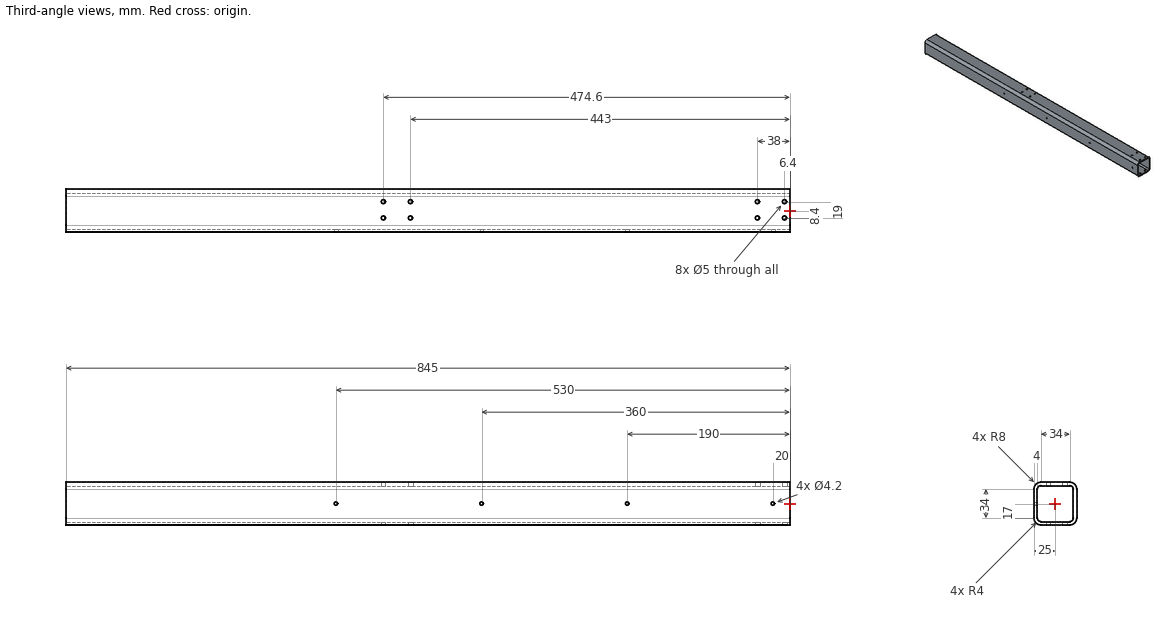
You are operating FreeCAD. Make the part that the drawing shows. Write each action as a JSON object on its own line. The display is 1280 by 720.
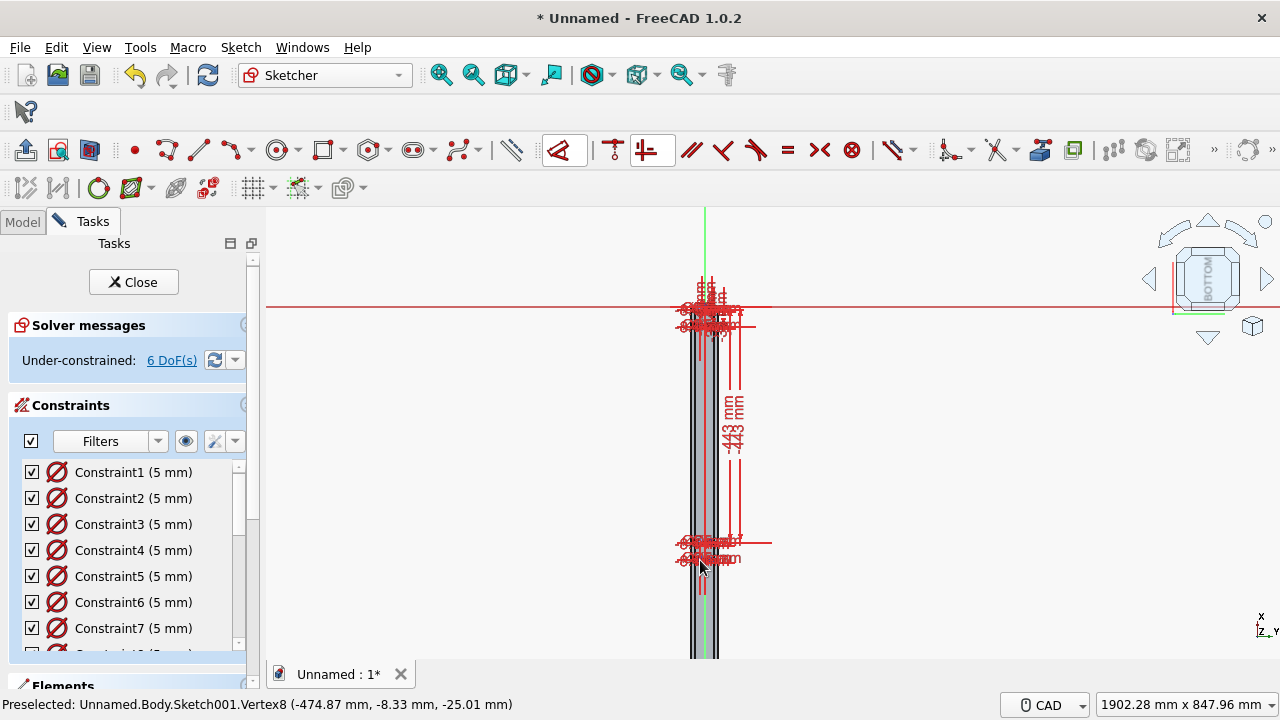
{"action": "scroll", "coordinate": [710, 310], "scroll_direction": "up", "scroll_amount": 7}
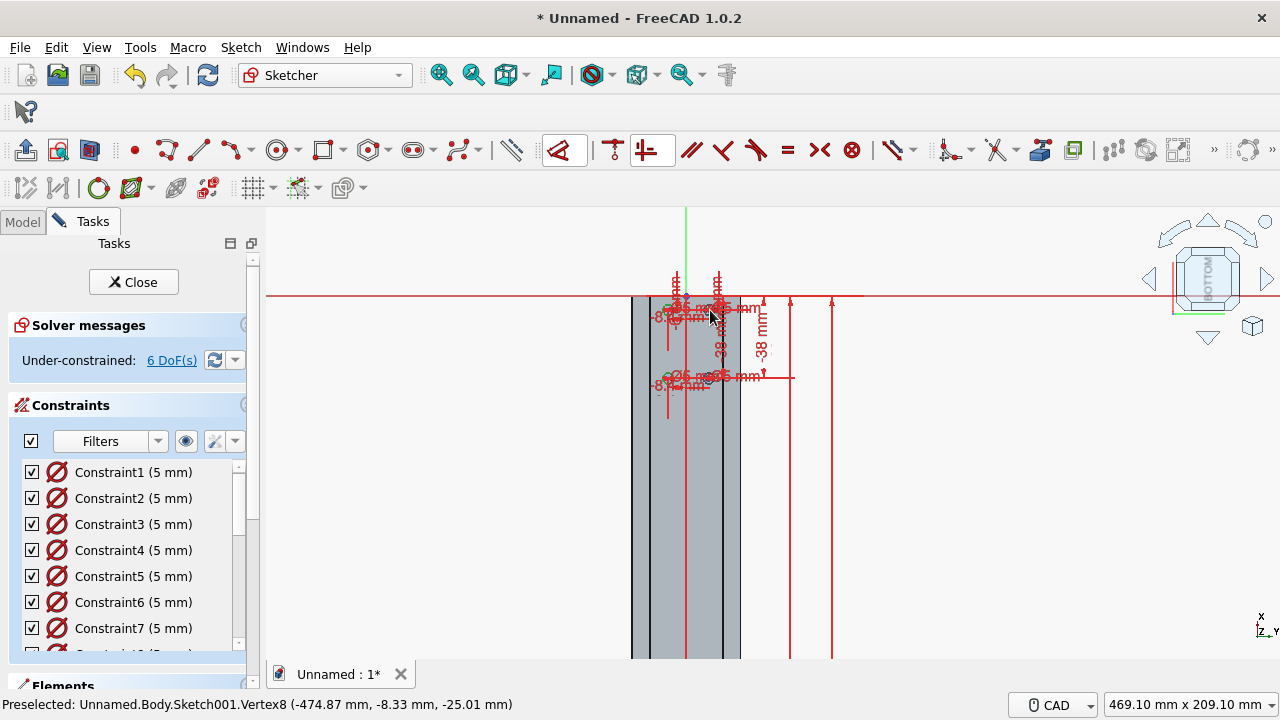
{"action": "left_click", "coordinate": [710, 310]}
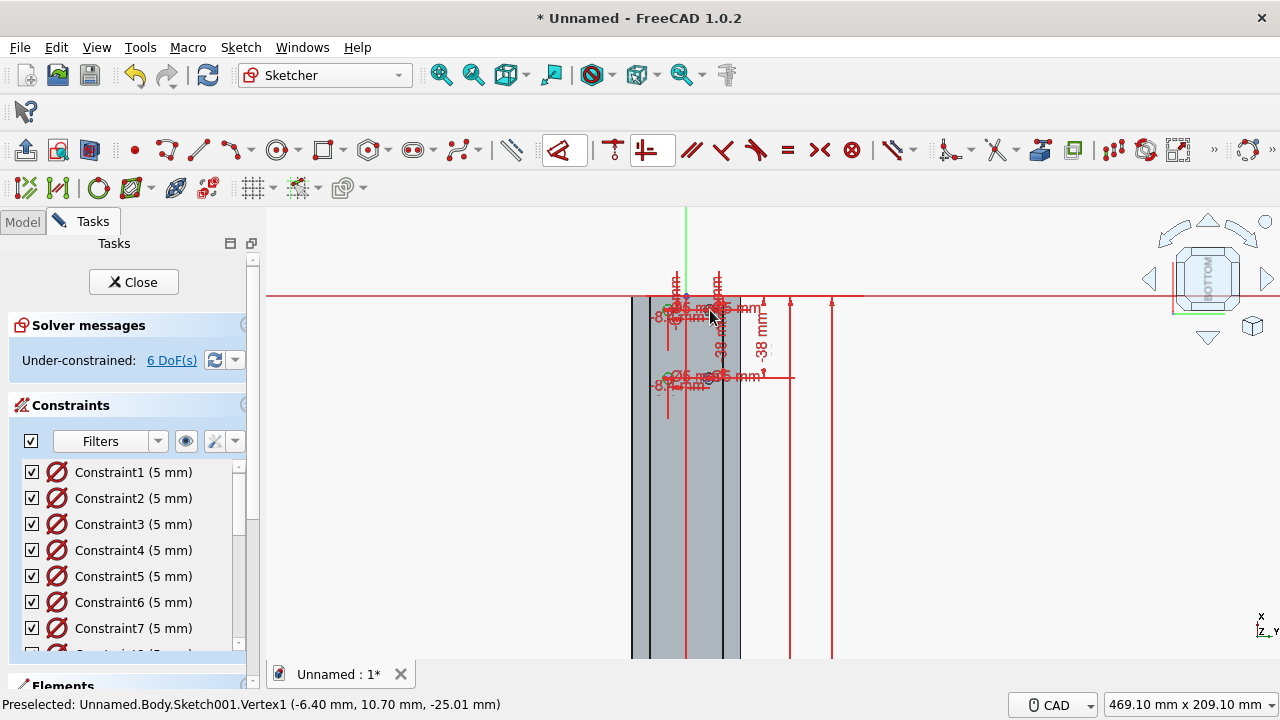
{"action": "left_click", "coordinate": [668, 310]}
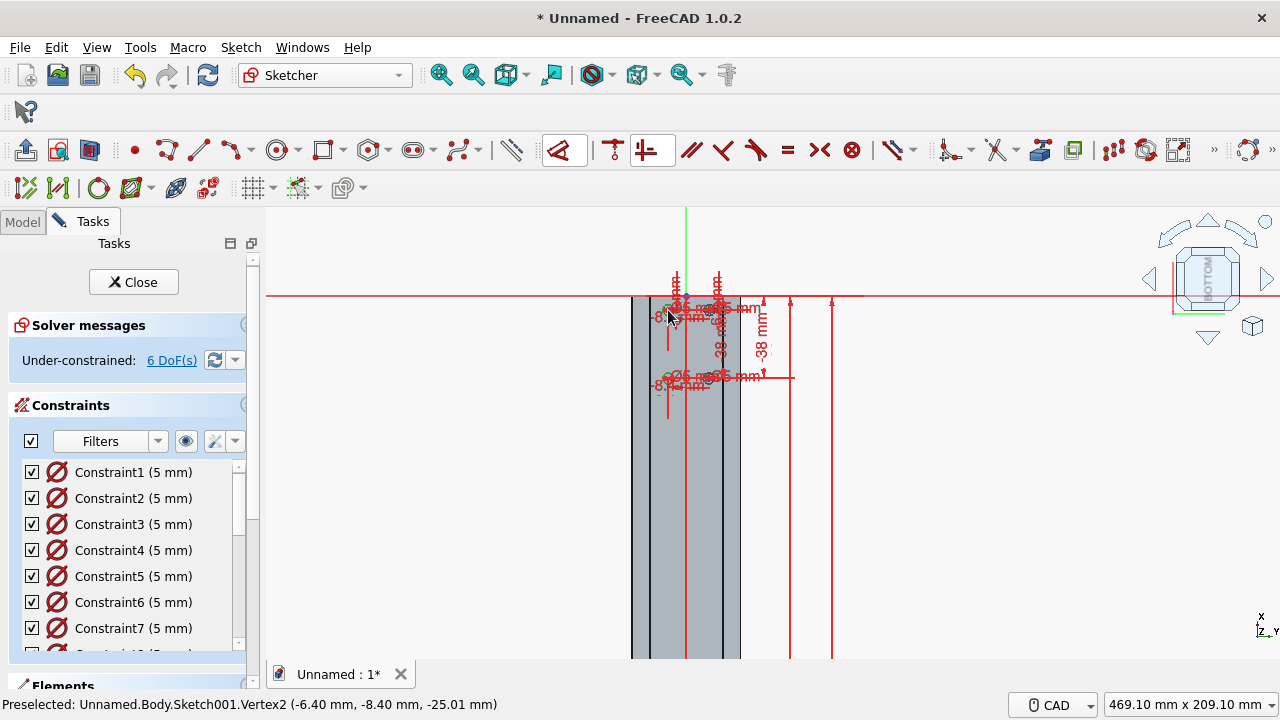
{"action": "left_click", "coordinate": [582, 150]}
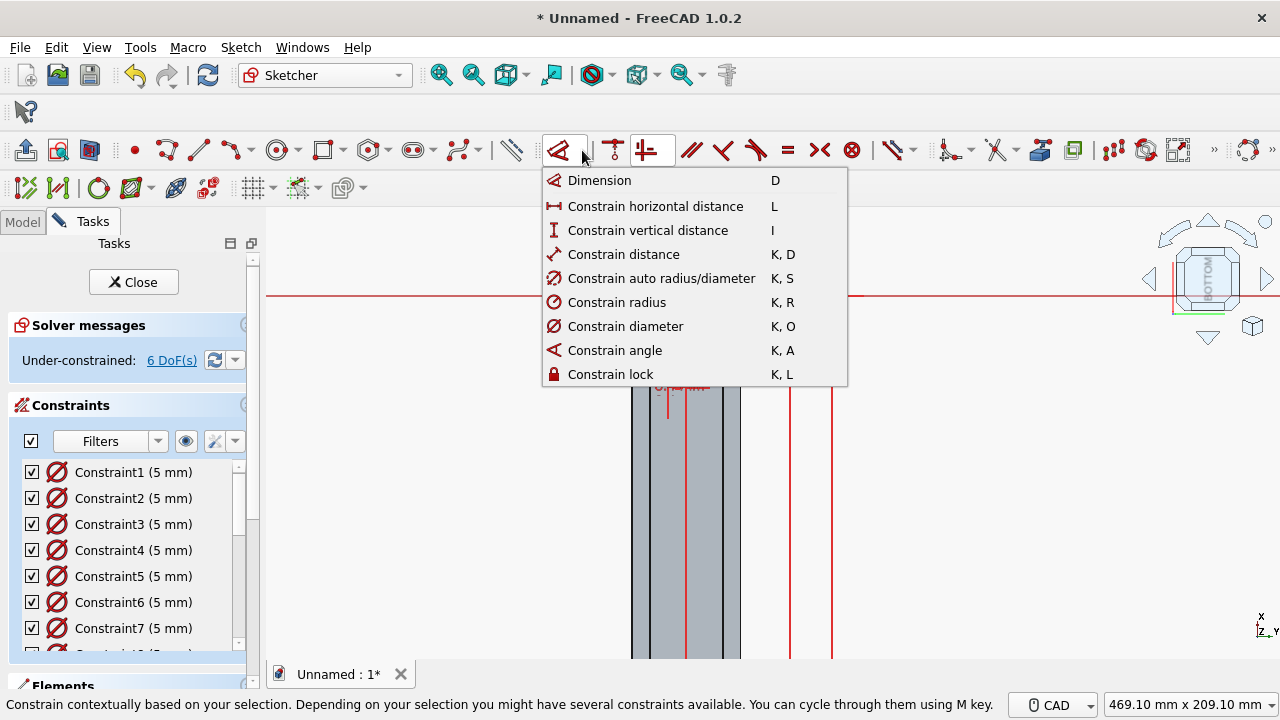
{"action": "left_click", "coordinate": [695, 206]}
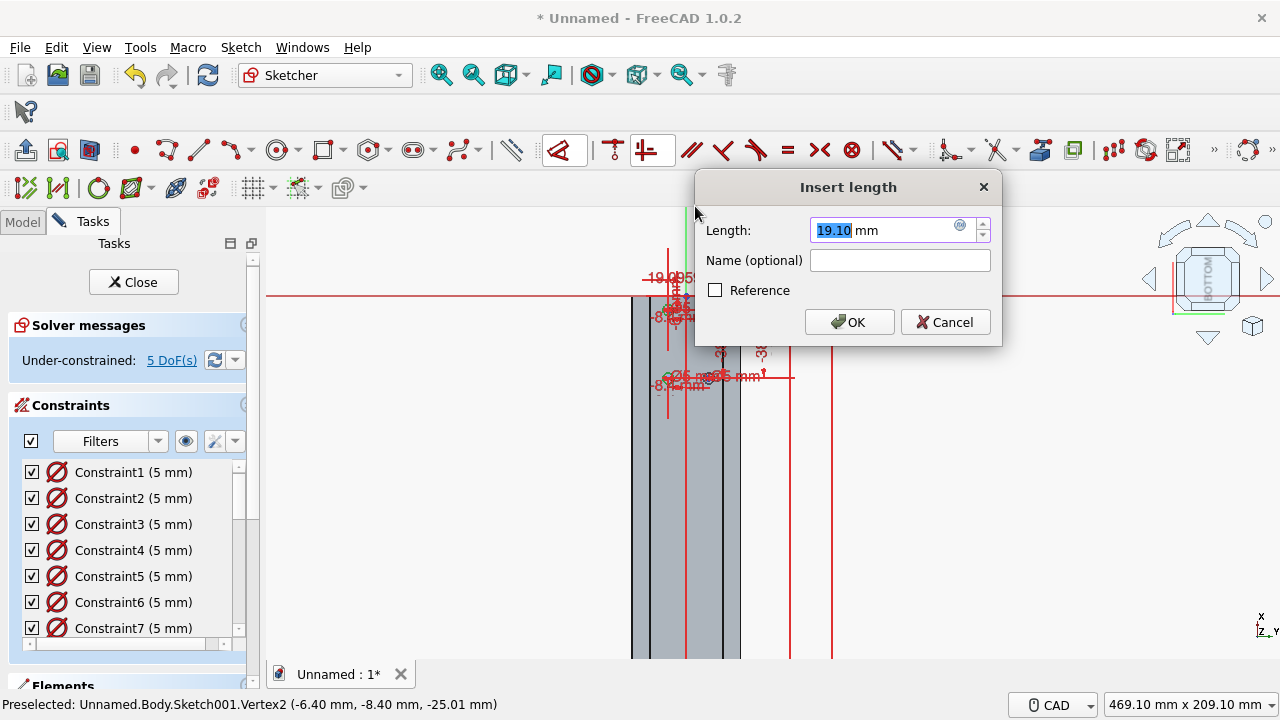
{"action": "type", "text": "19"}
{"action": "key", "text": "Return"}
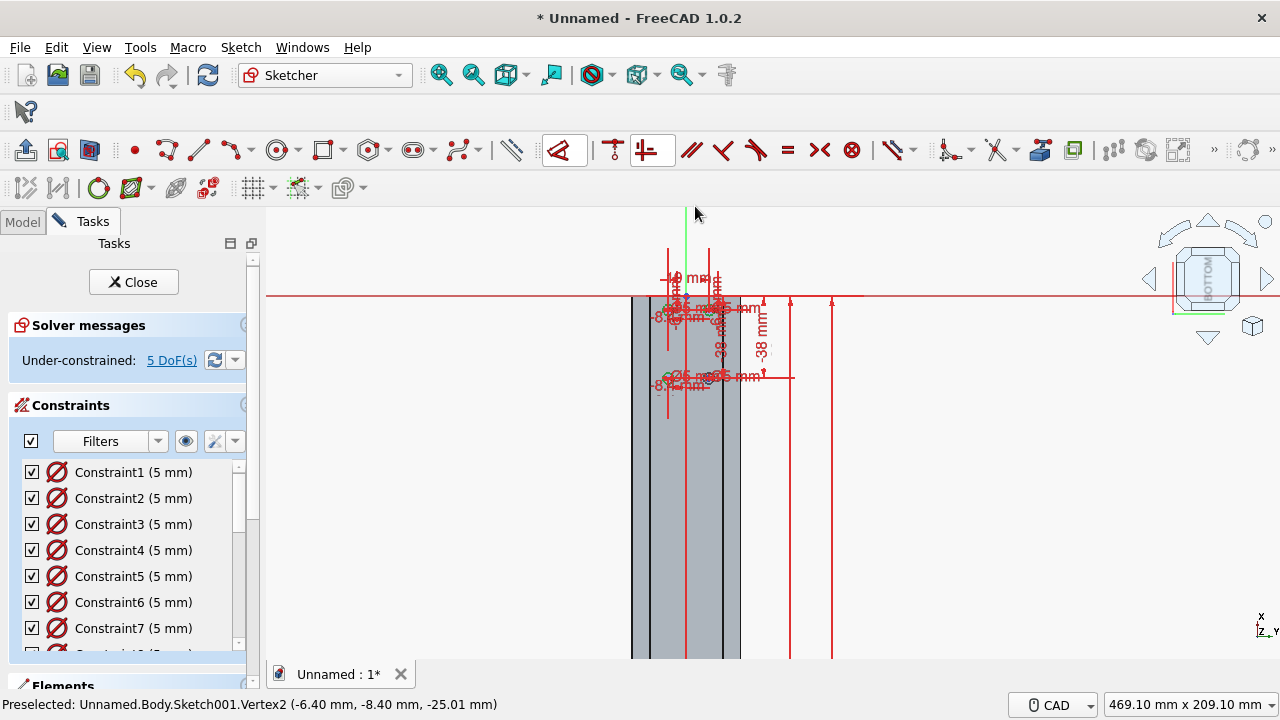
{"action": "left_click", "coordinate": [668, 310]}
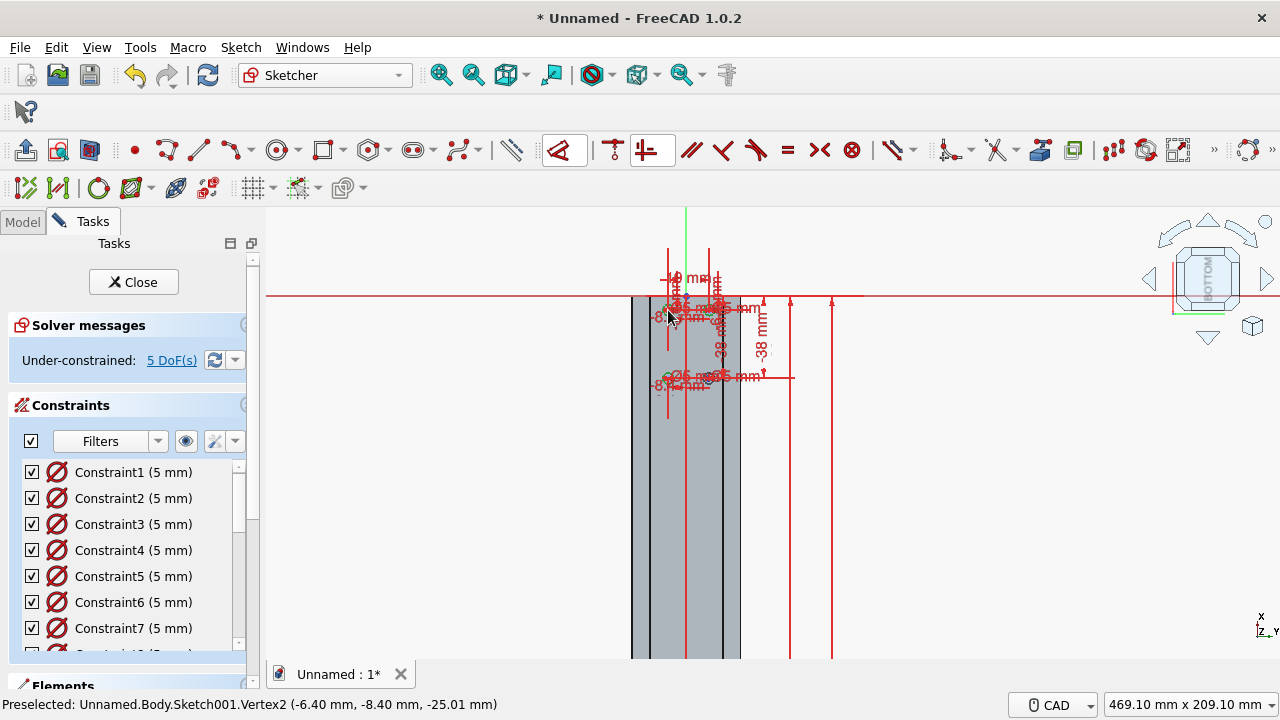
{"action": "left_click", "coordinate": [709, 378]}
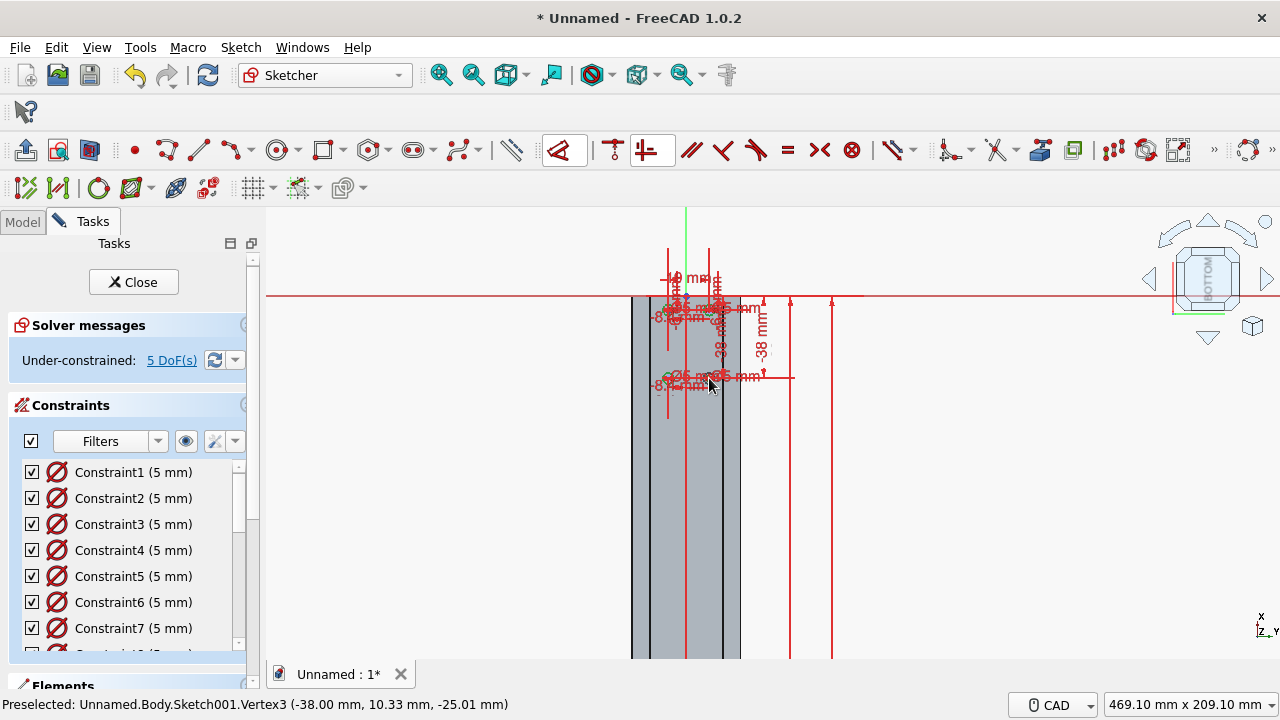
{"action": "left_click", "coordinate": [582, 150]}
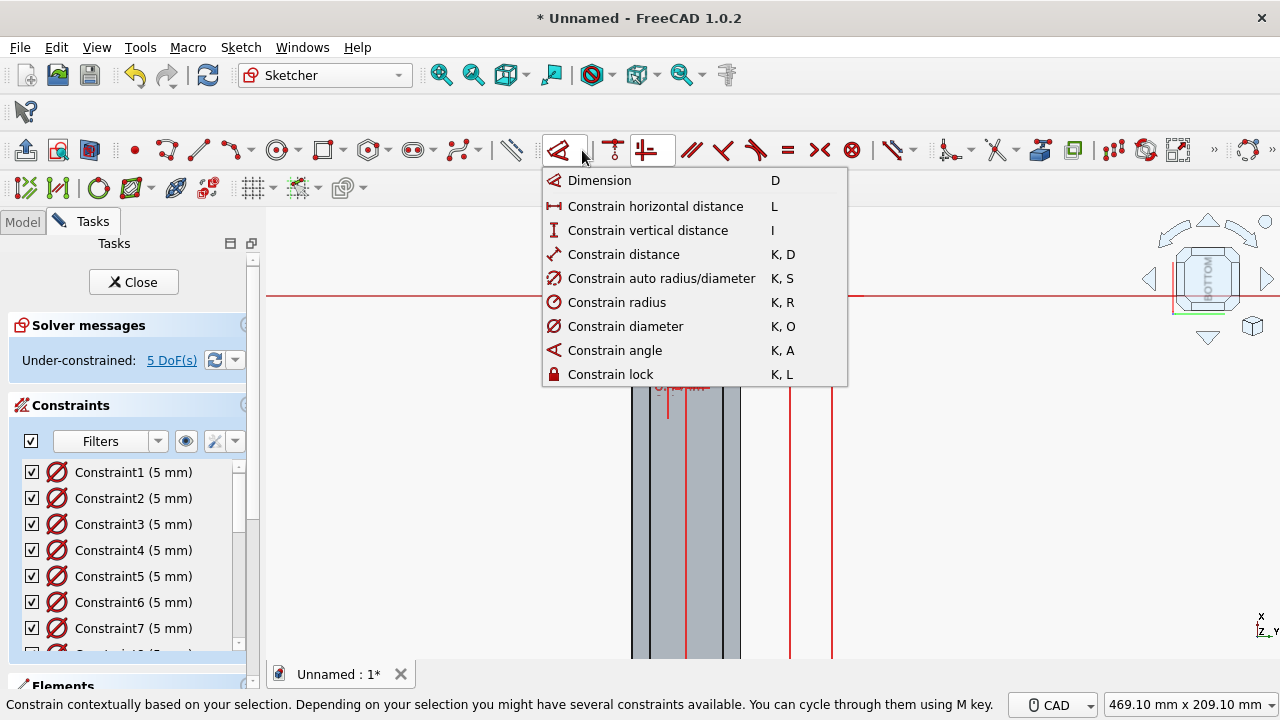
{"action": "left_click", "coordinate": [695, 206]}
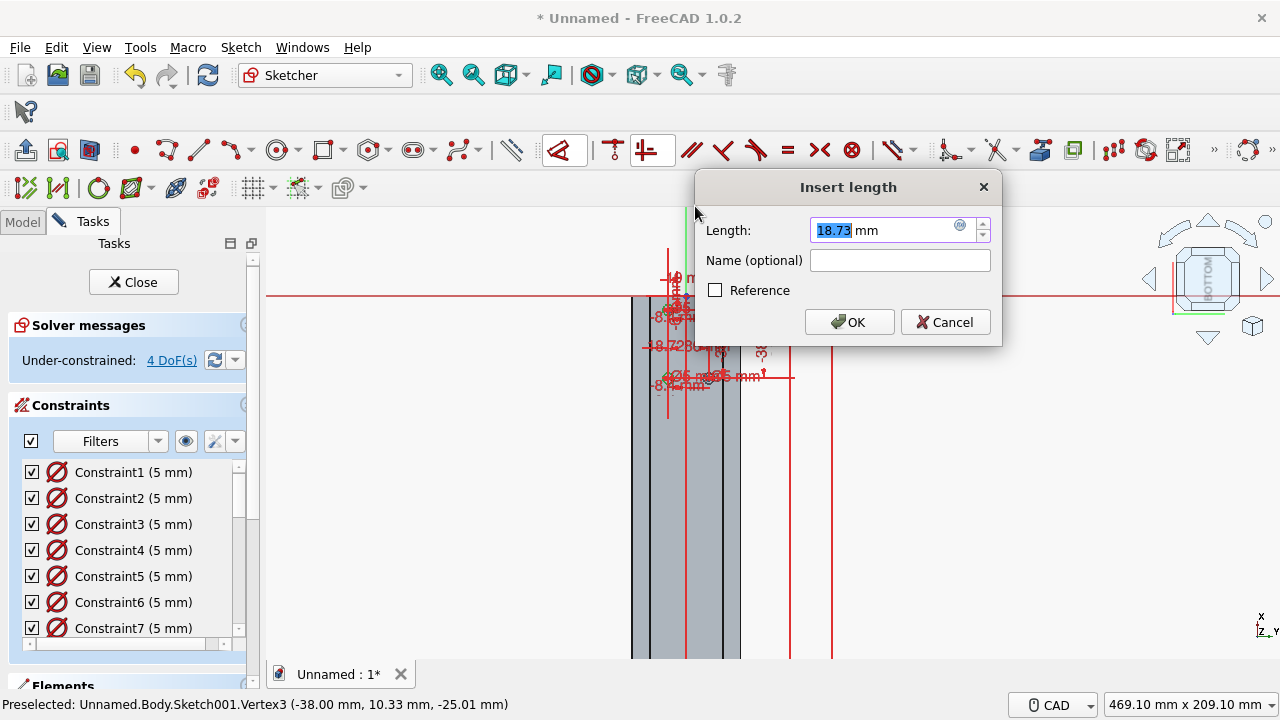
{"action": "type", "text": "19"}
{"action": "key", "text": "Return"}